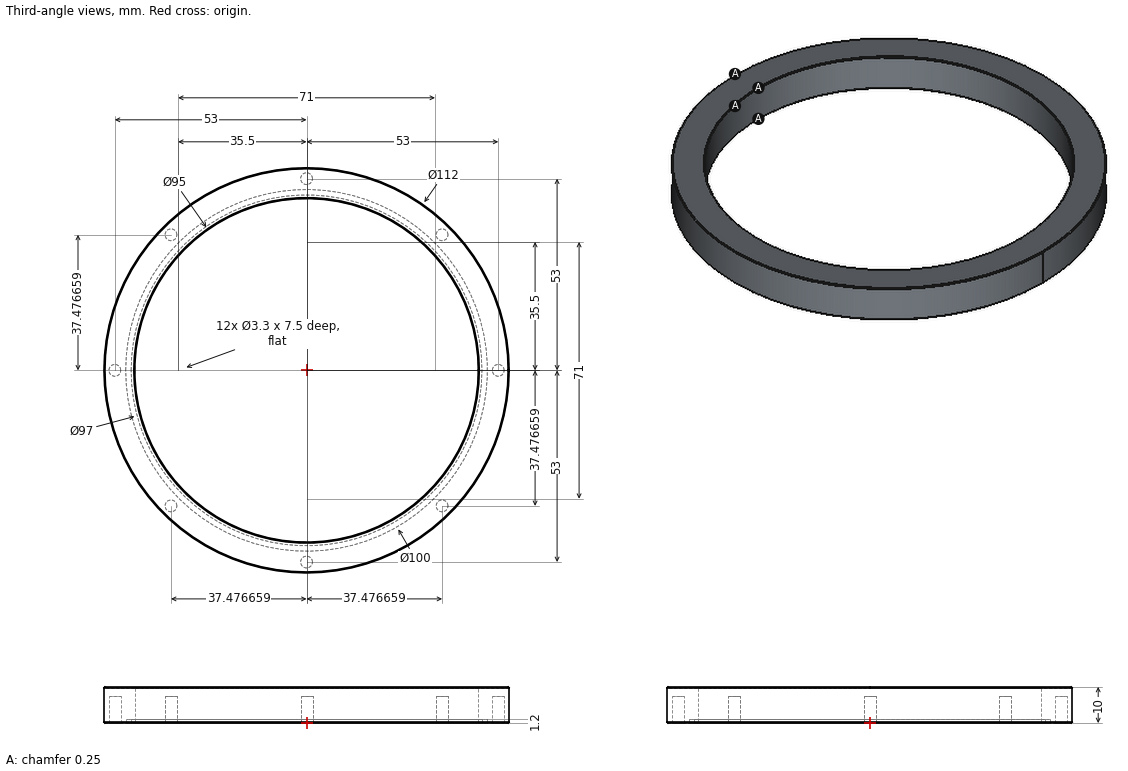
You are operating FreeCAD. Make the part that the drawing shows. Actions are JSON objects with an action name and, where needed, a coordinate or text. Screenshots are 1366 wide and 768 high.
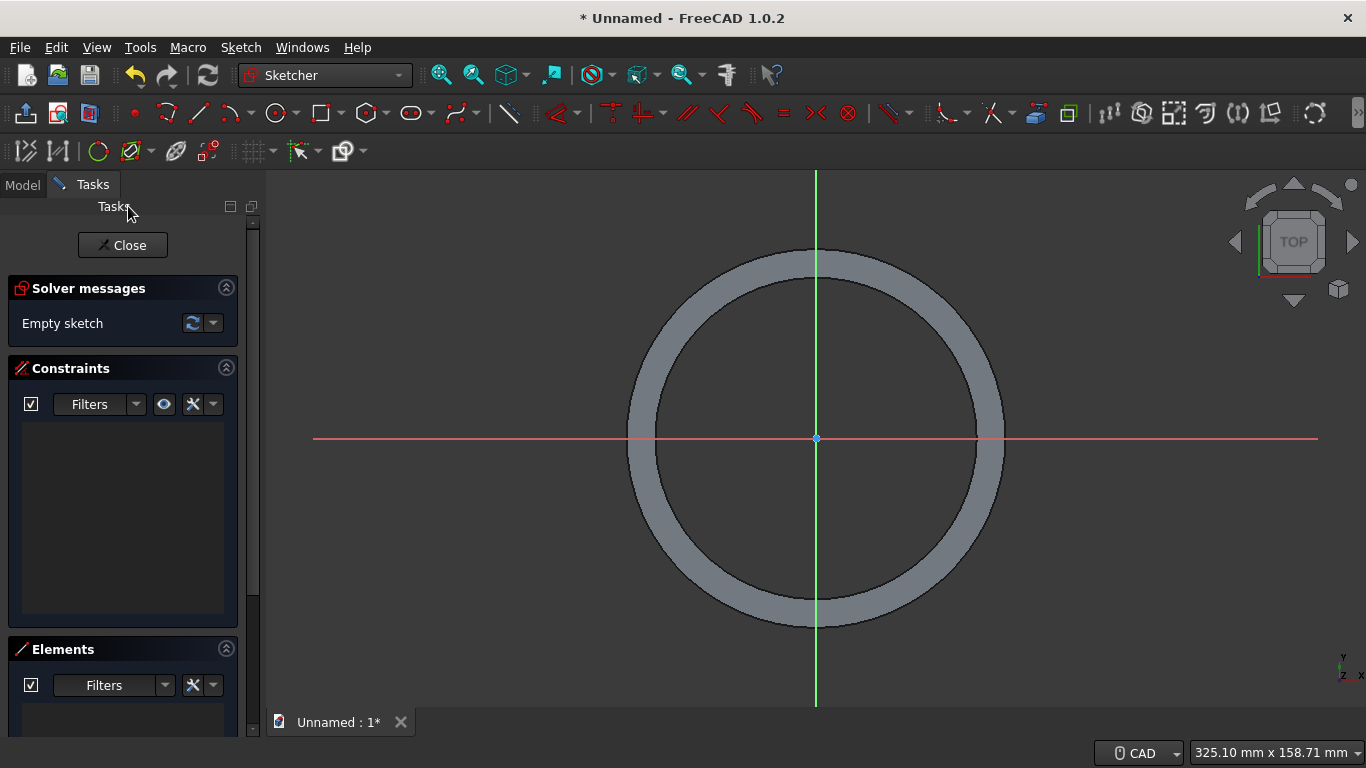
{"action": "left_click", "coordinate": [276, 114]}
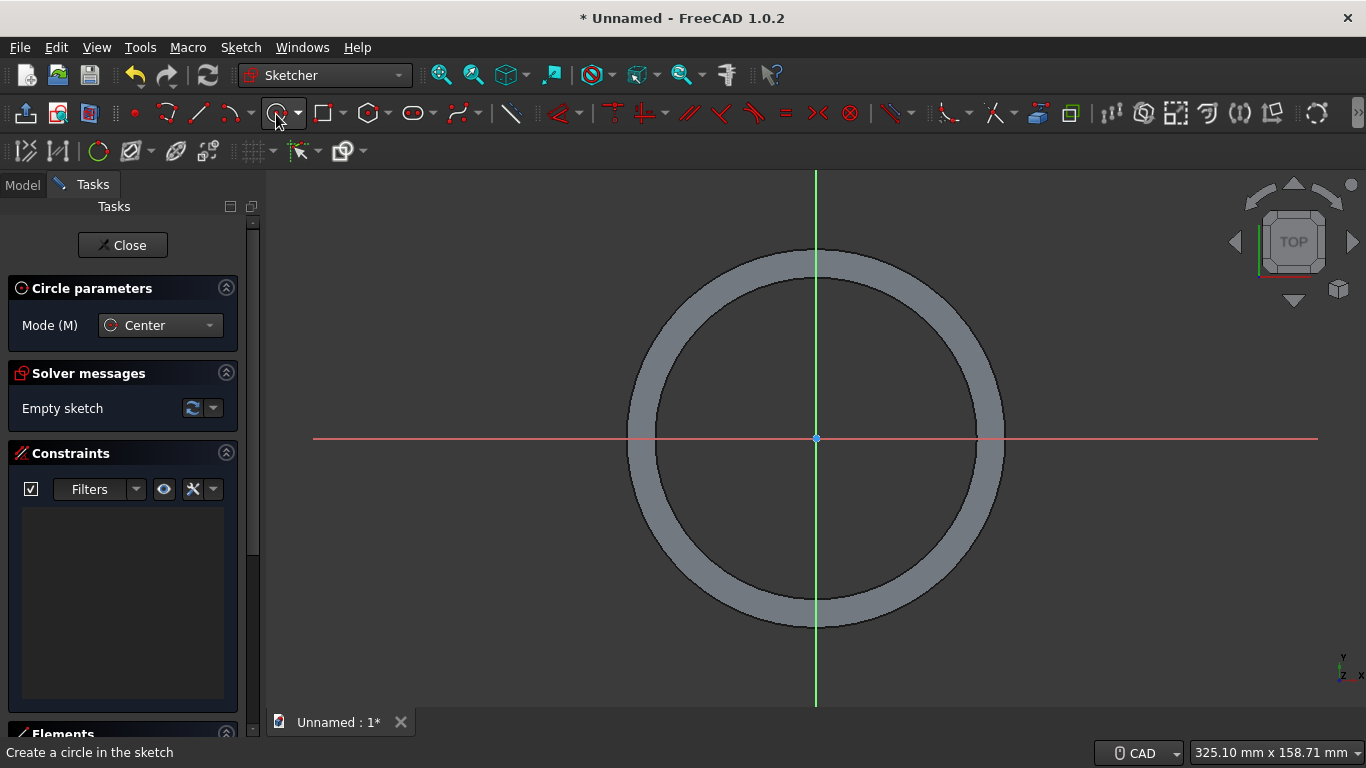
{"action": "scroll", "coordinate": [696, 438], "scroll_direction": "up", "scroll_amount": 8}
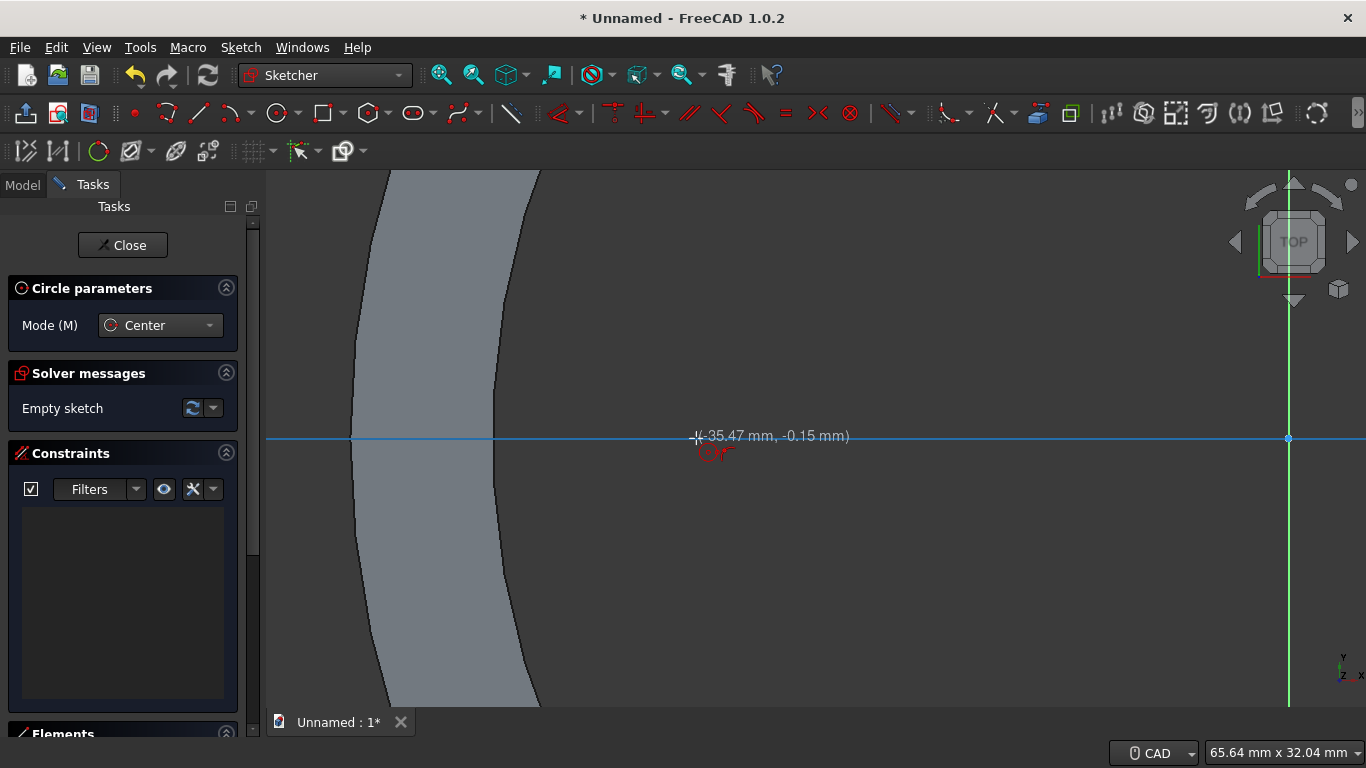
{"action": "scroll", "coordinate": [611, 438], "scroll_direction": "down", "scroll_amount": 8}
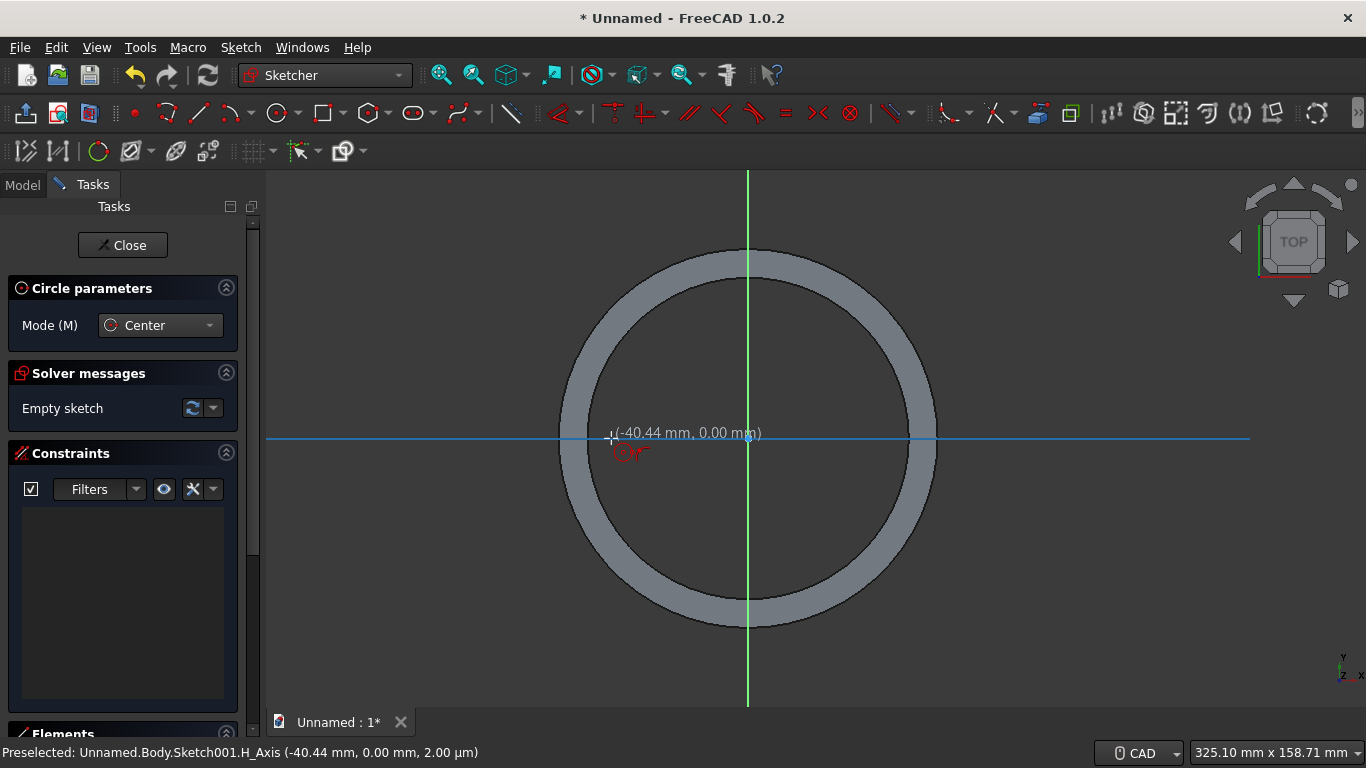
{"action": "left_click", "coordinate": [628, 438]}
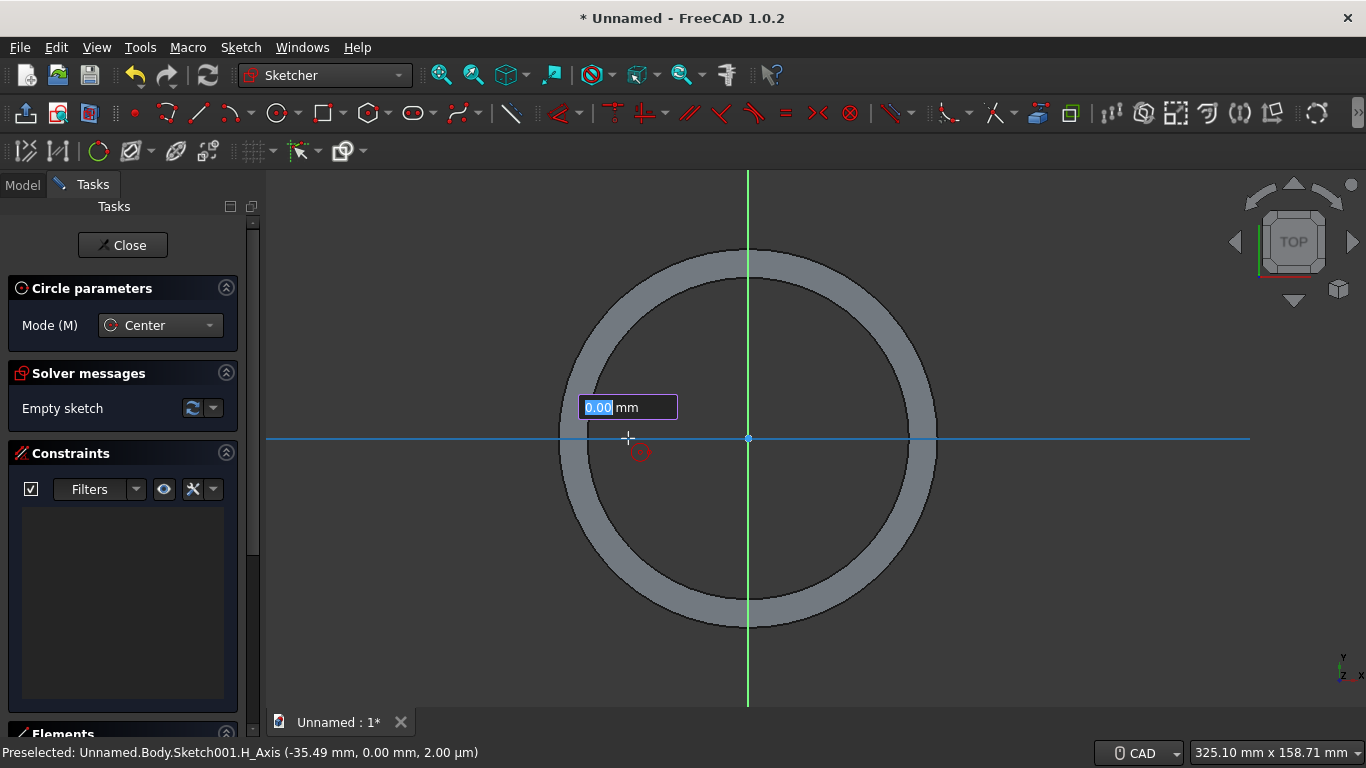
{"action": "scroll", "coordinate": [626, 444], "scroll_direction": "up", "scroll_amount": 6}
{"action": "mouse_move", "coordinate": [625, 442]}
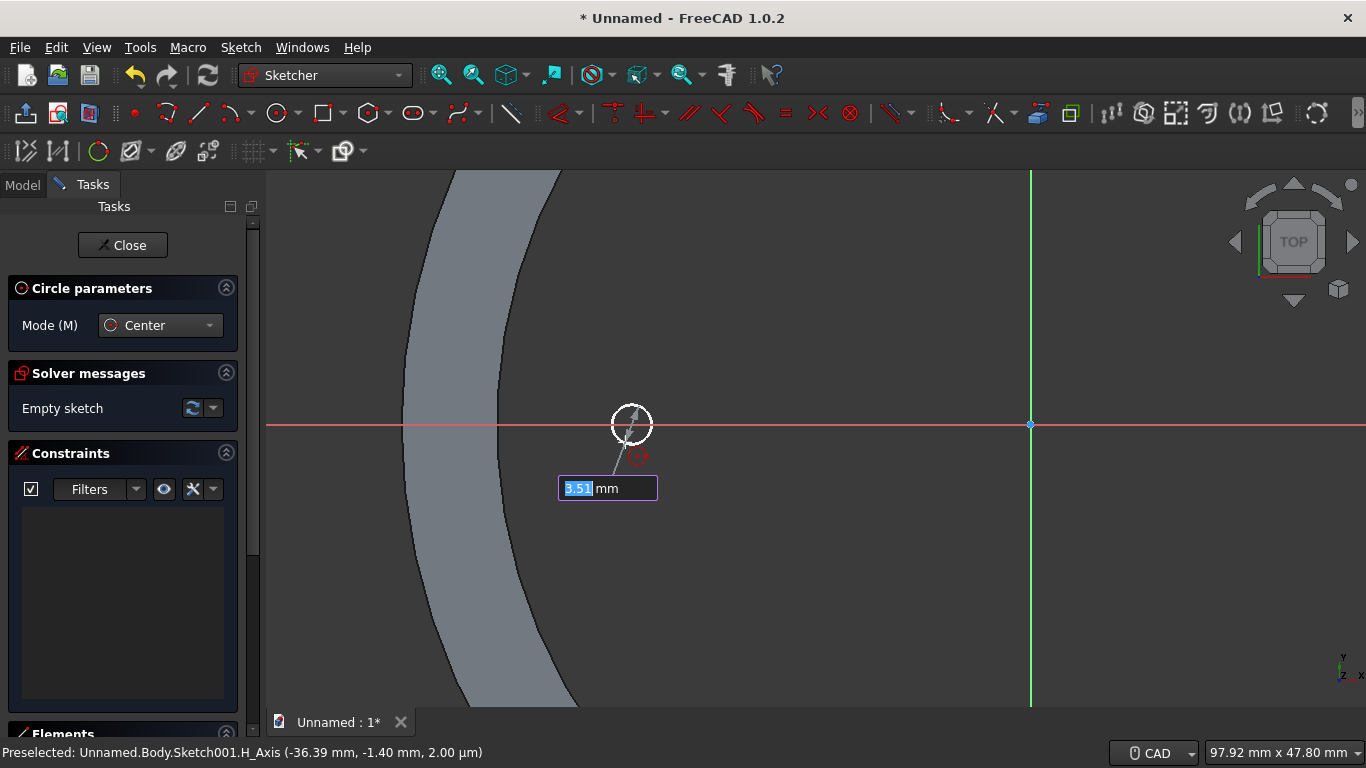
{"action": "type", "text": "3.3"}
{"action": "key", "text": "Return"}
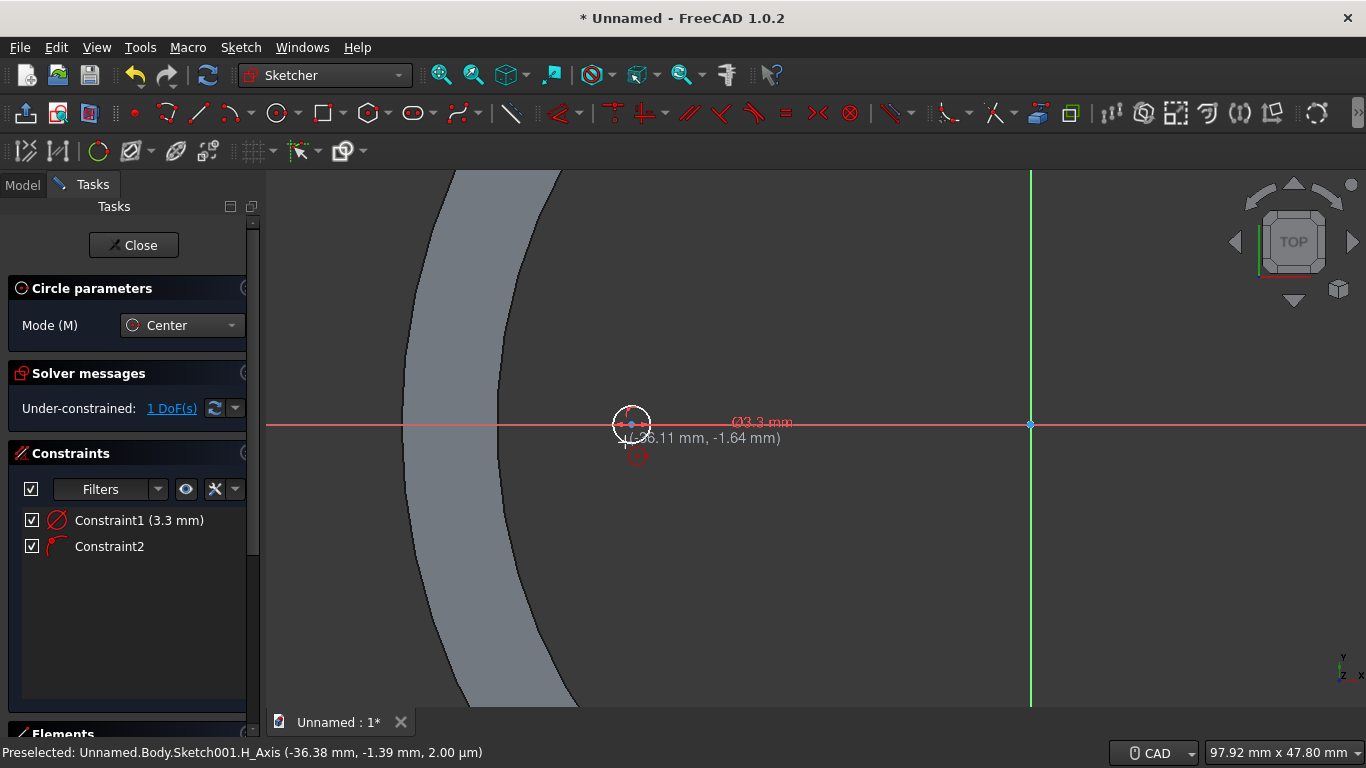
{"action": "scroll", "coordinate": [625, 445], "scroll_direction": "down", "scroll_amount": 6}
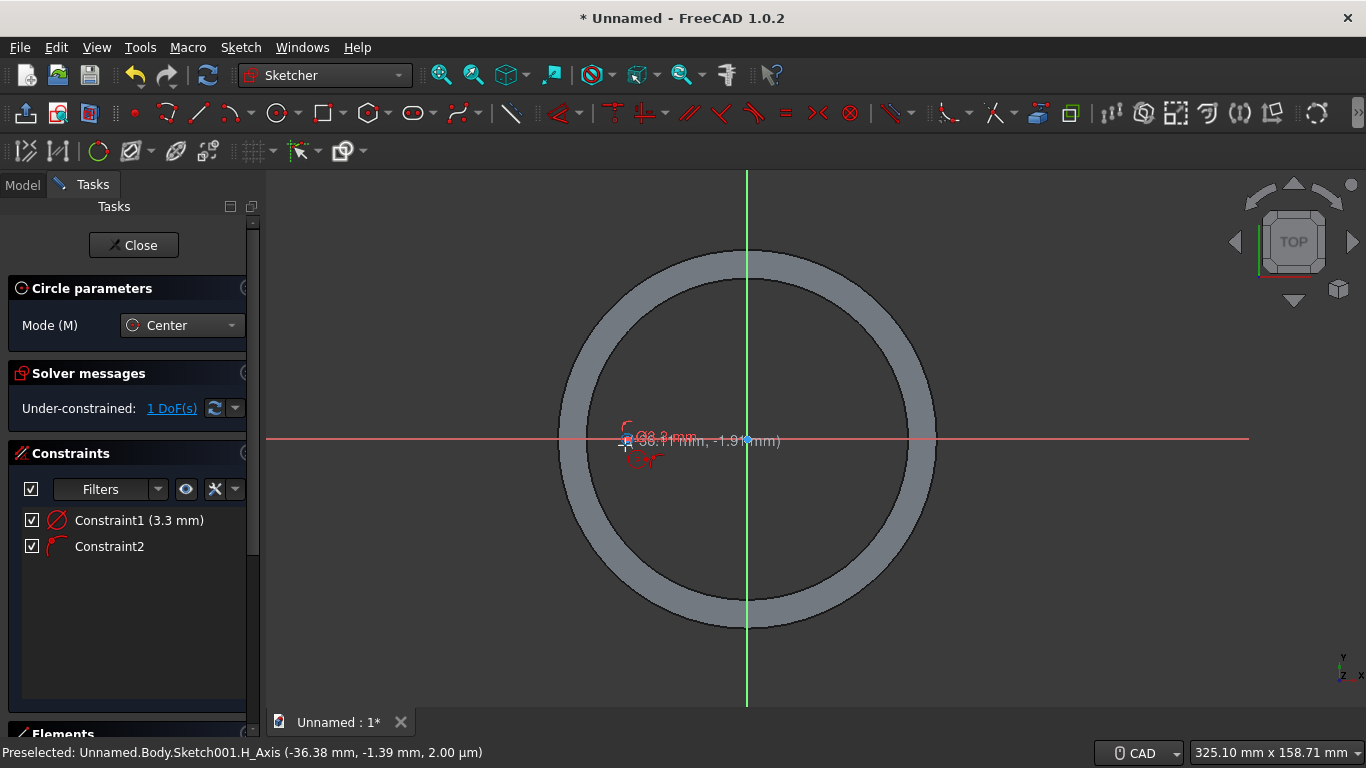
{"action": "scroll", "coordinate": [747, 319], "scroll_direction": "up", "scroll_amount": 8}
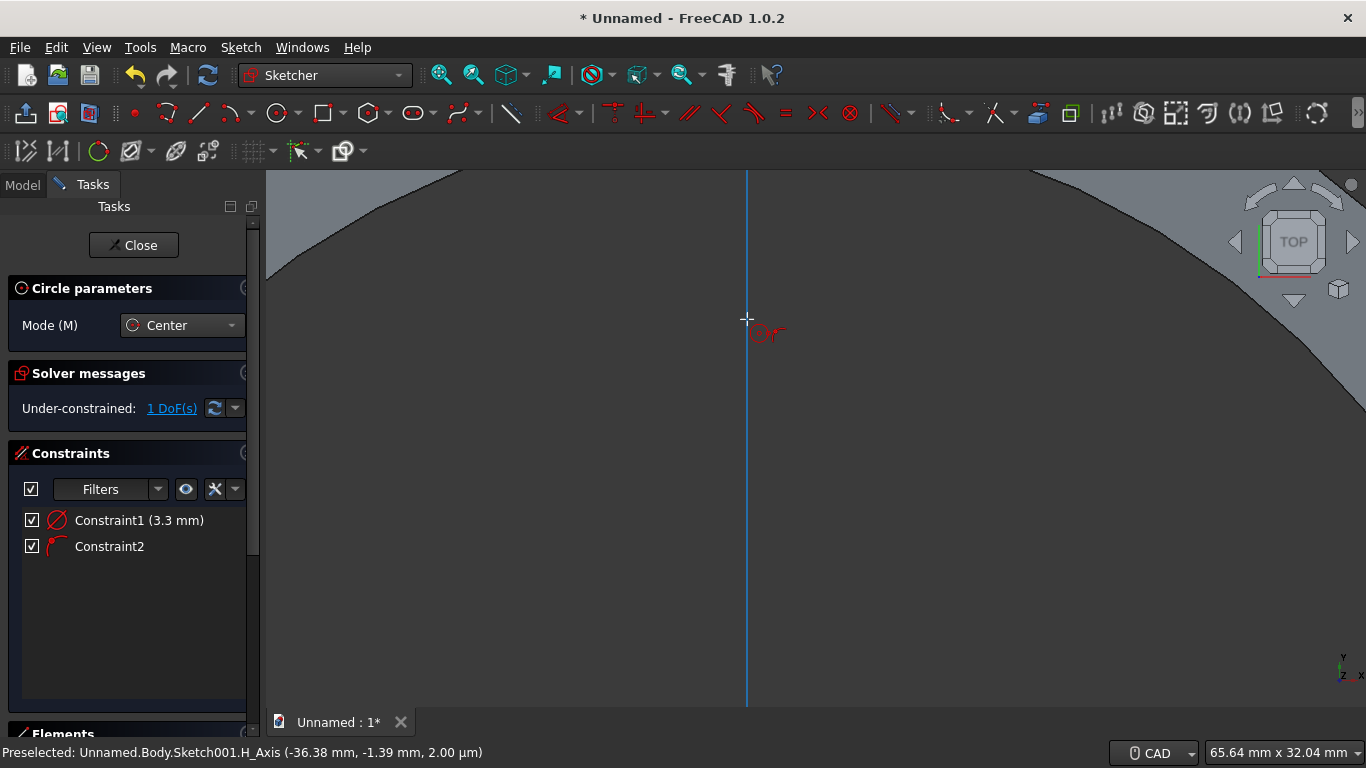
{"action": "scroll", "coordinate": [748, 318], "scroll_direction": "down", "scroll_amount": 8}